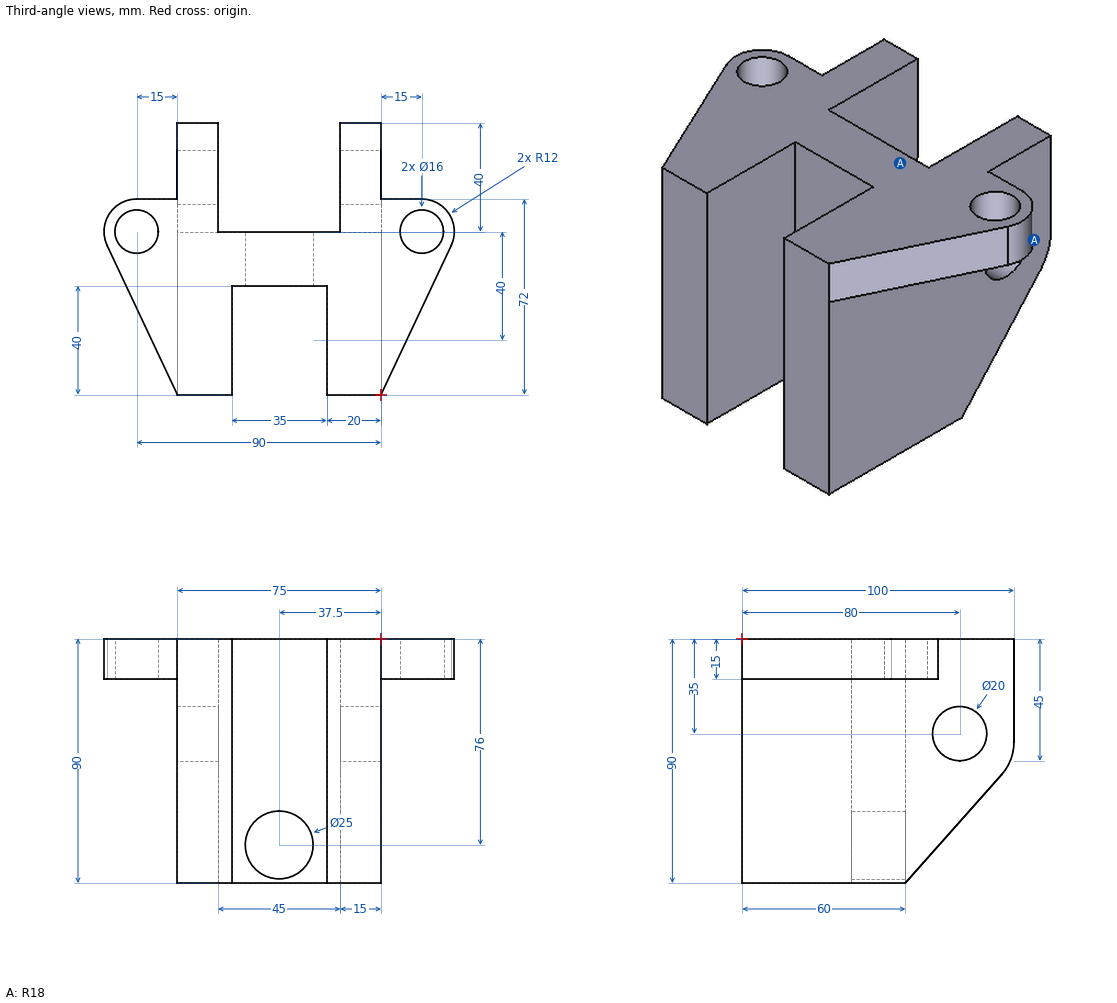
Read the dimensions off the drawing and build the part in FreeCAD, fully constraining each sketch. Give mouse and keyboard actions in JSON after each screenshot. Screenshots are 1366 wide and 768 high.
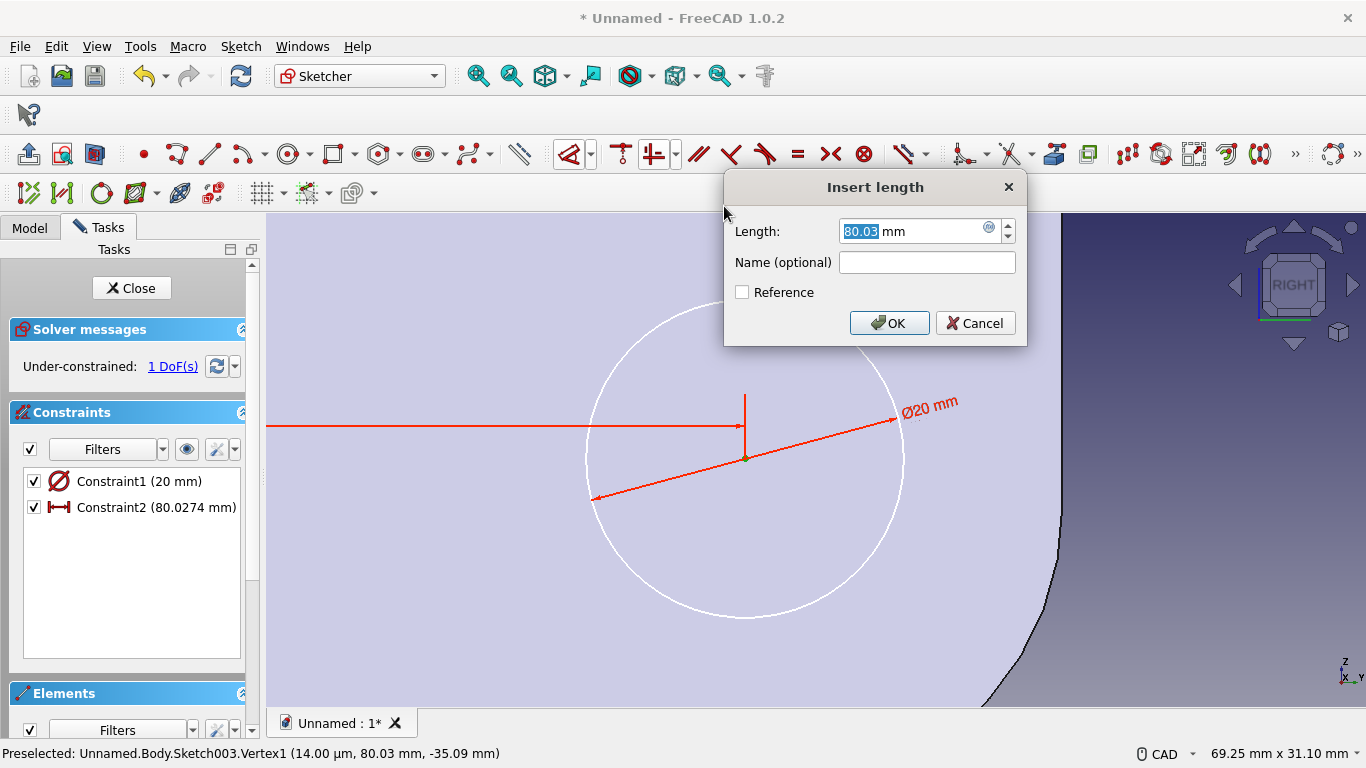
{"action": "type", "text": "80"}
{"action": "key", "text": "Return"}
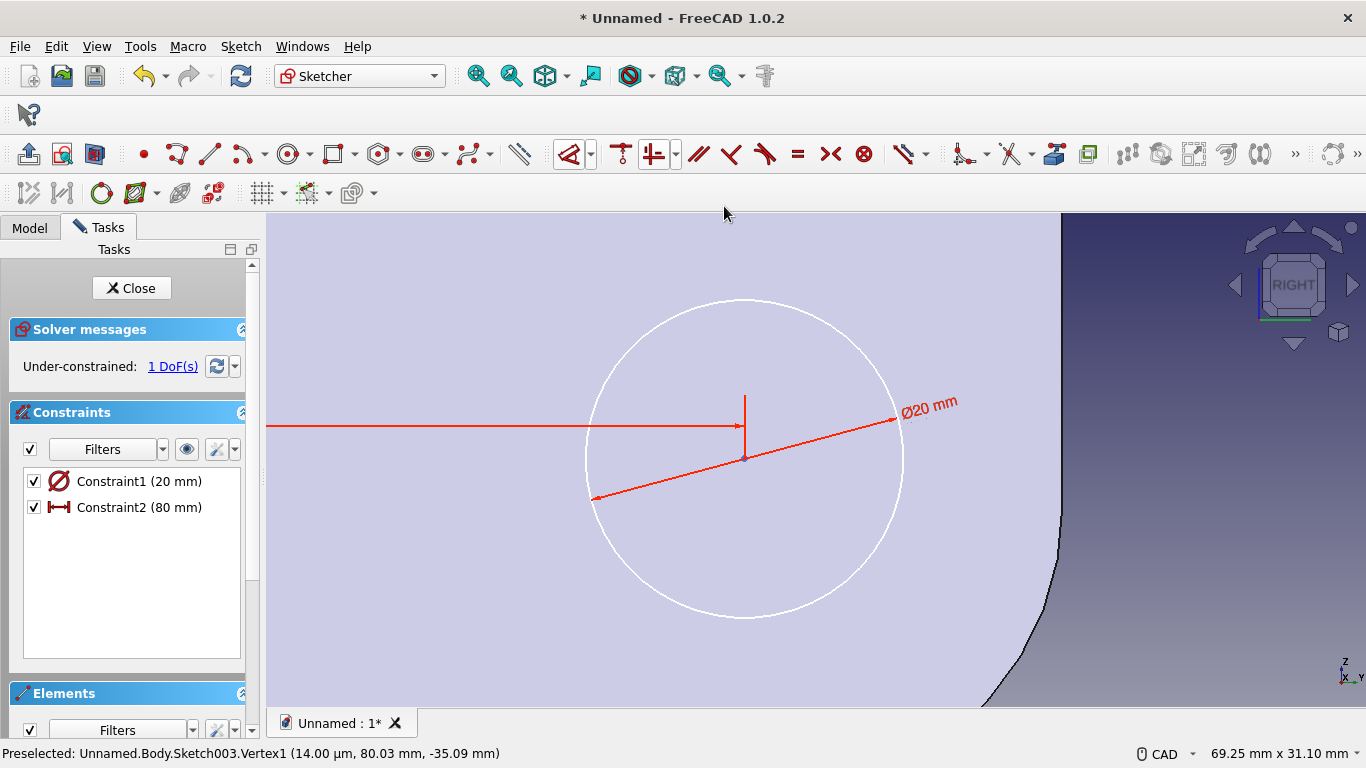
{"action": "left_click", "coordinate": [745, 459]}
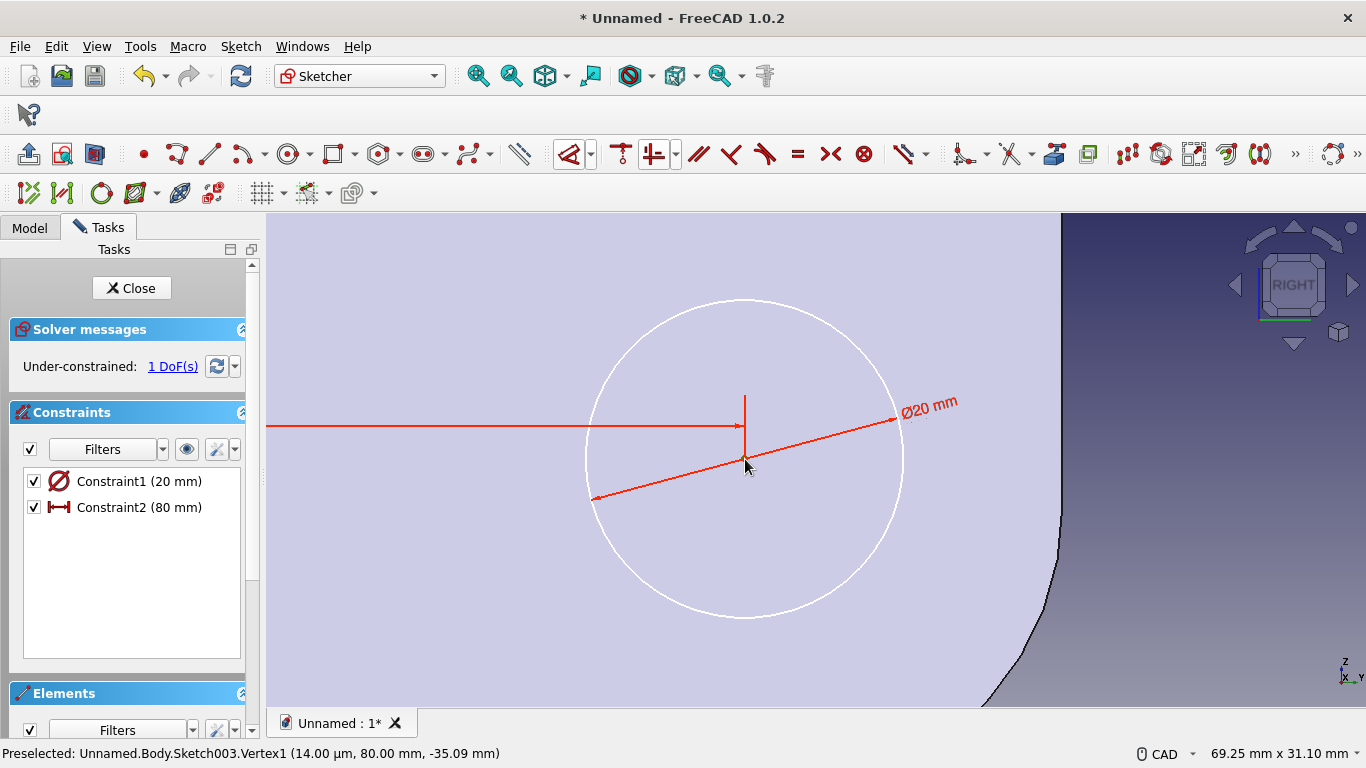
{"action": "key", "text": "i"}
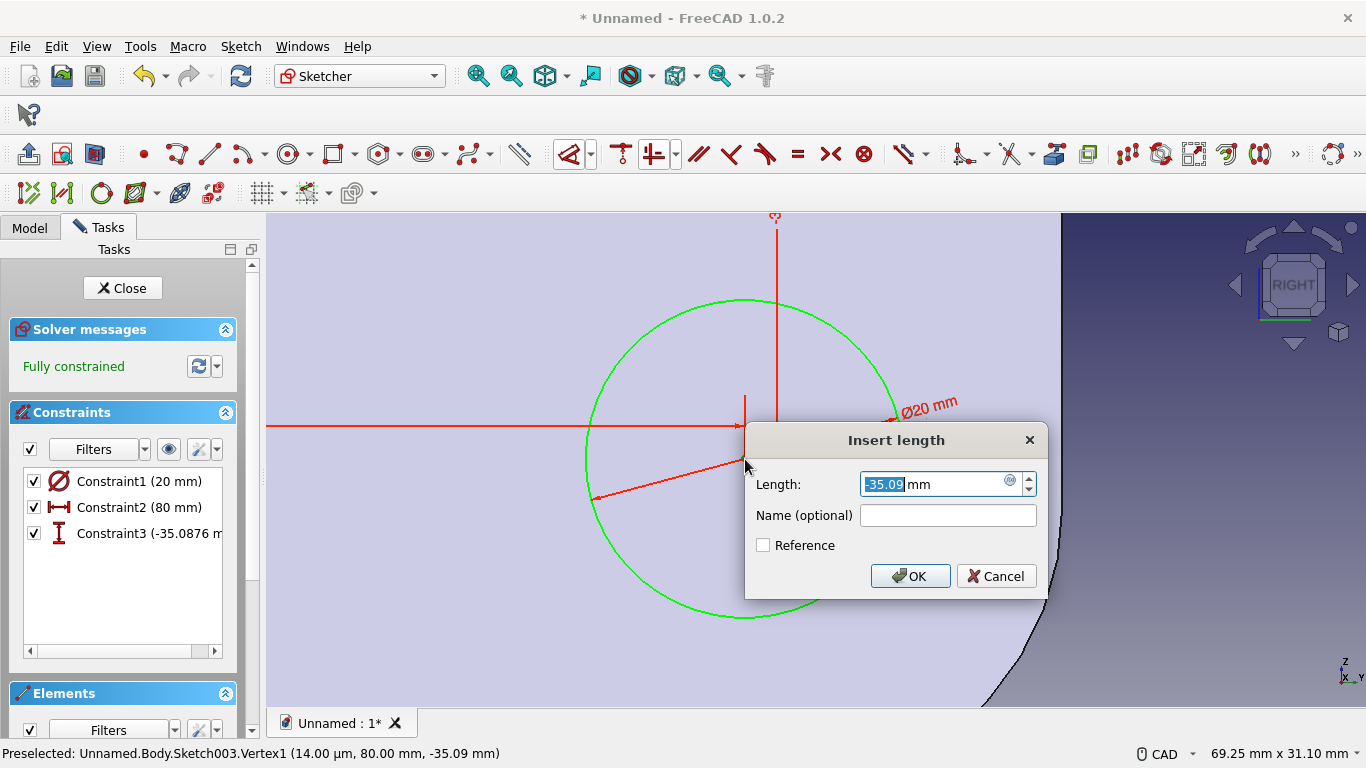
{"action": "type", "text": "-35"}
{"action": "key", "text": "Return"}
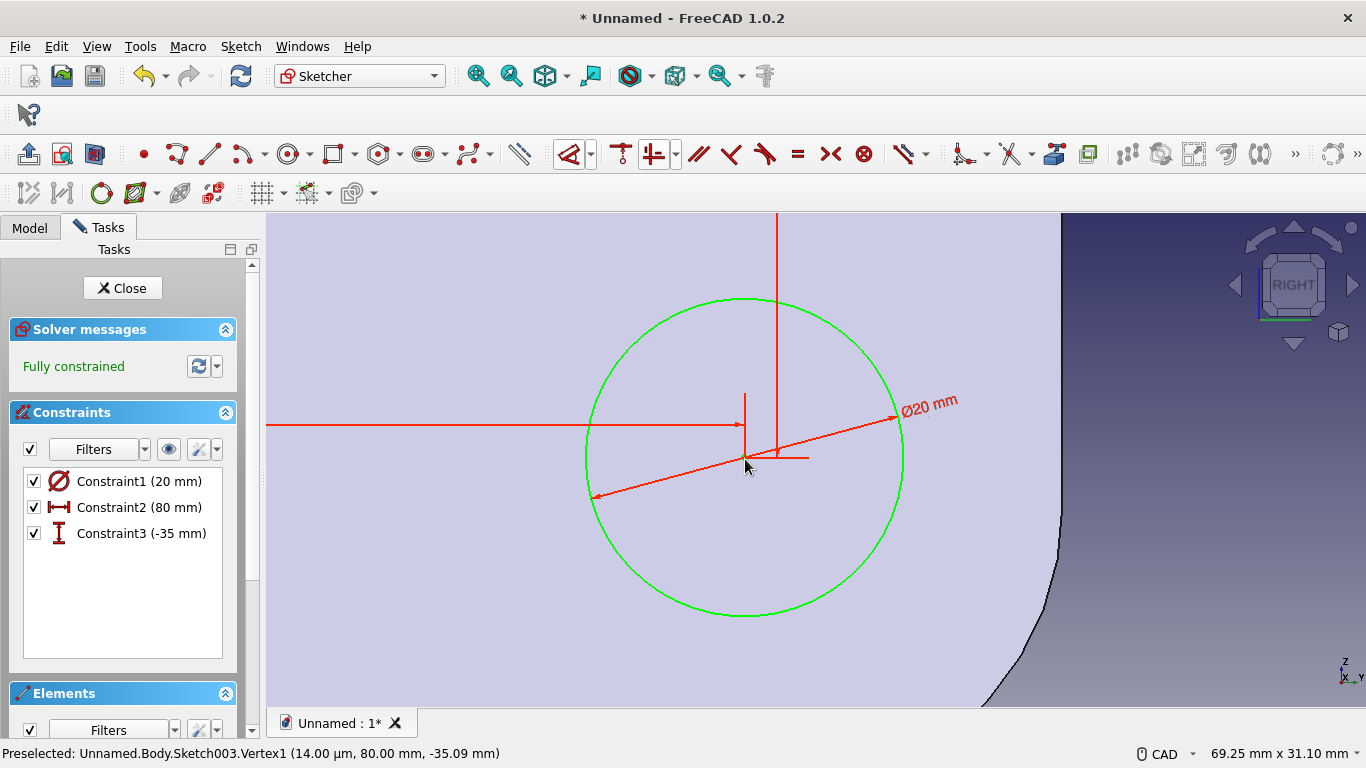
{"action": "left_click", "coordinate": [123, 288]}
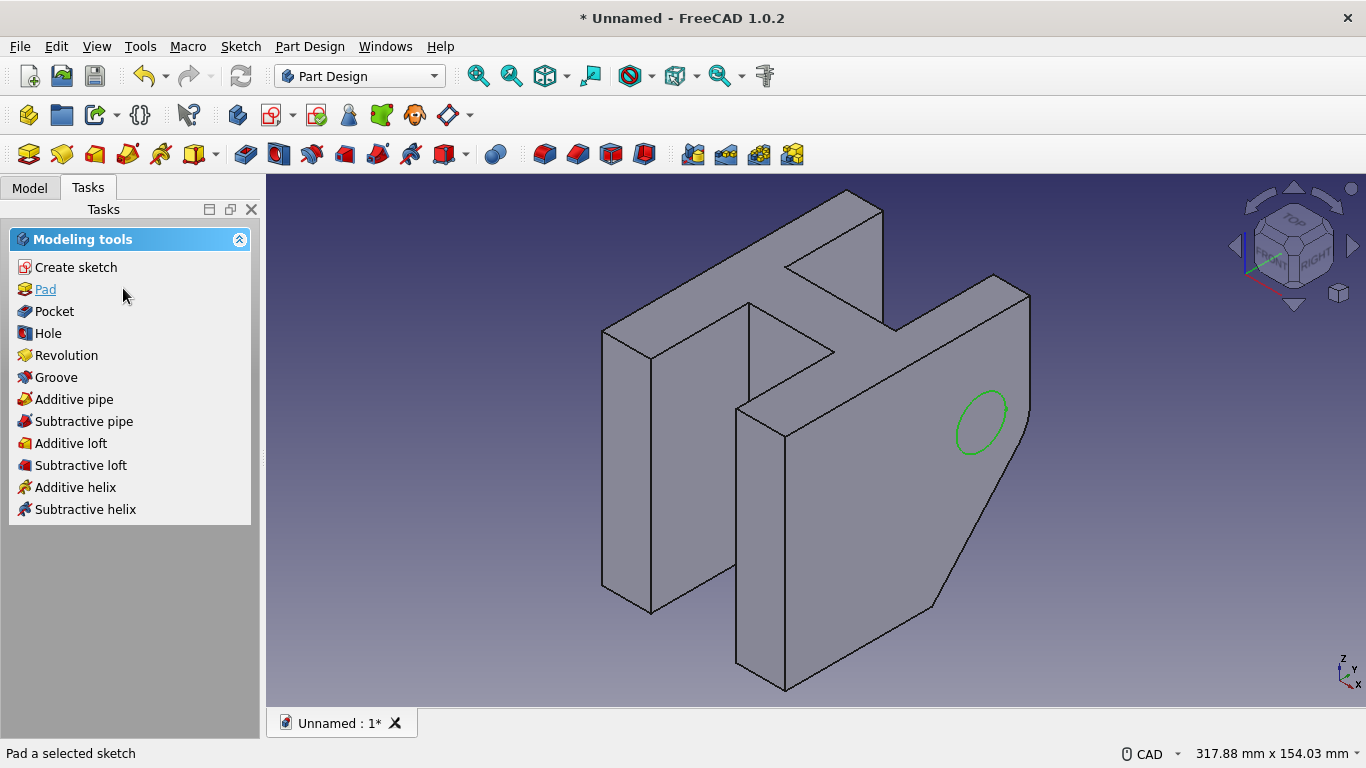
{"action": "left_click", "coordinate": [246, 154]}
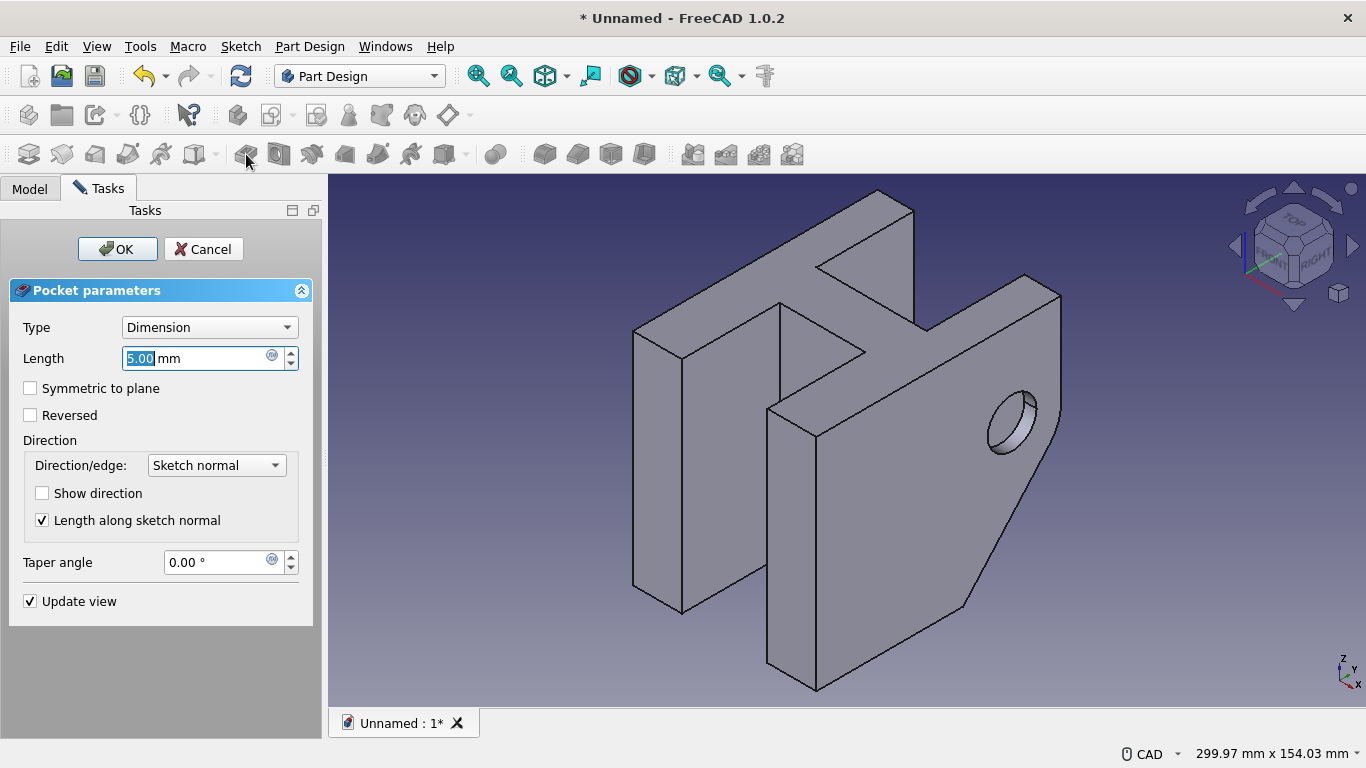
{"action": "left_click", "coordinate": [210, 328]}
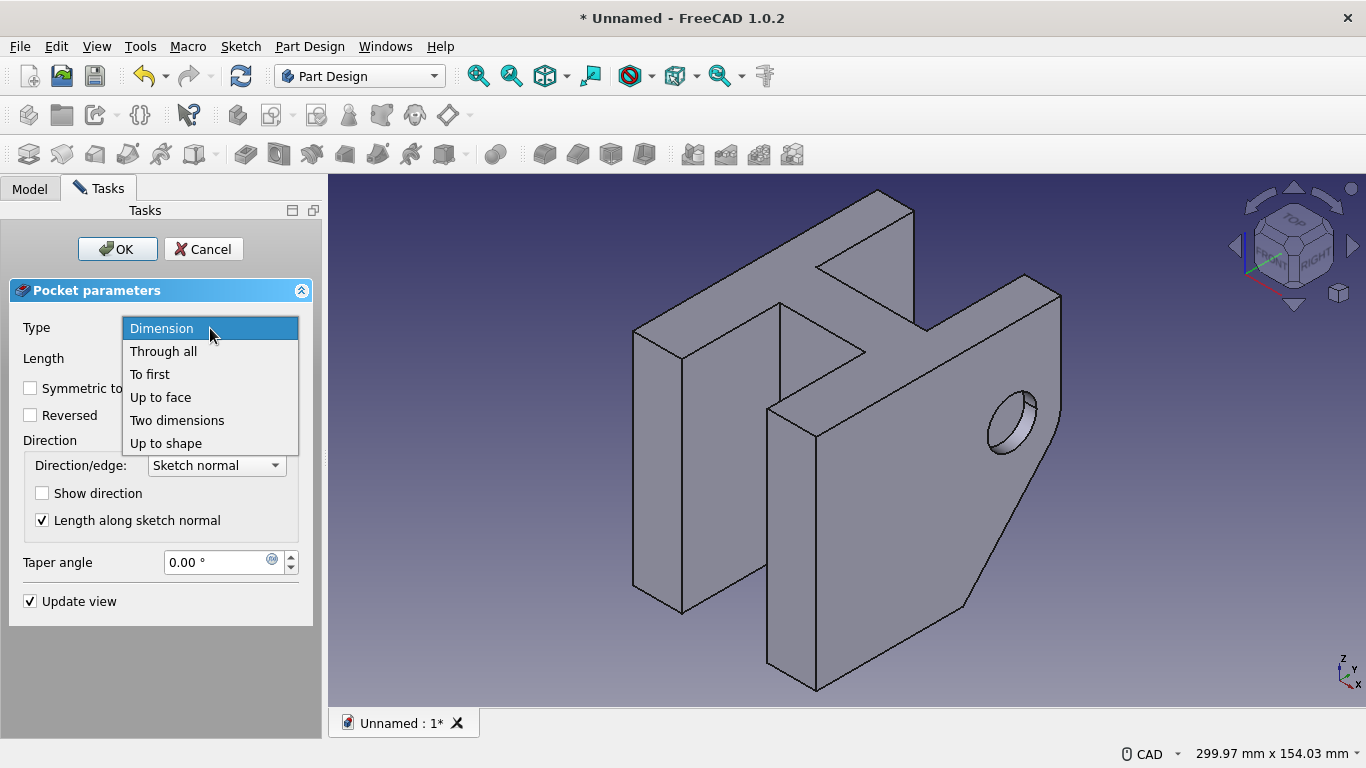
{"action": "left_click", "coordinate": [208, 352]}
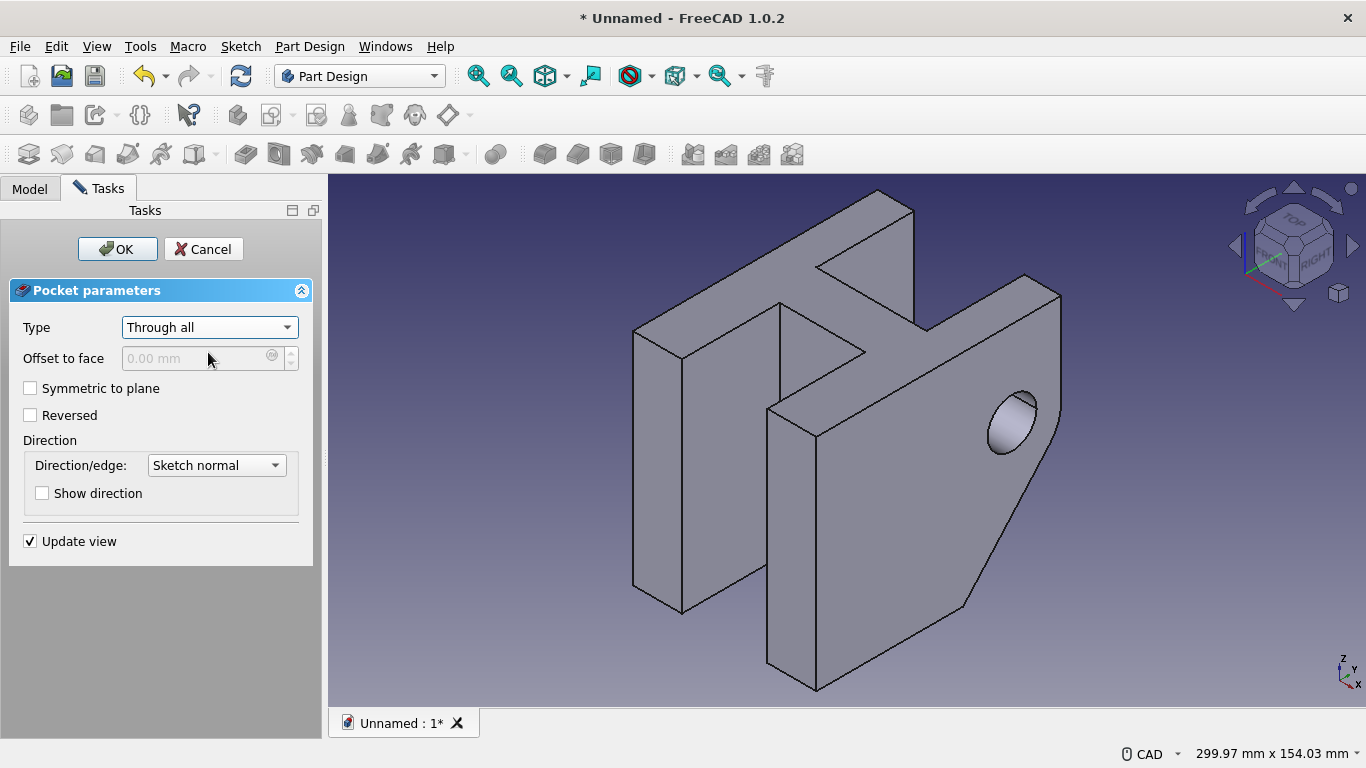
{"action": "left_click", "coordinate": [118, 249]}